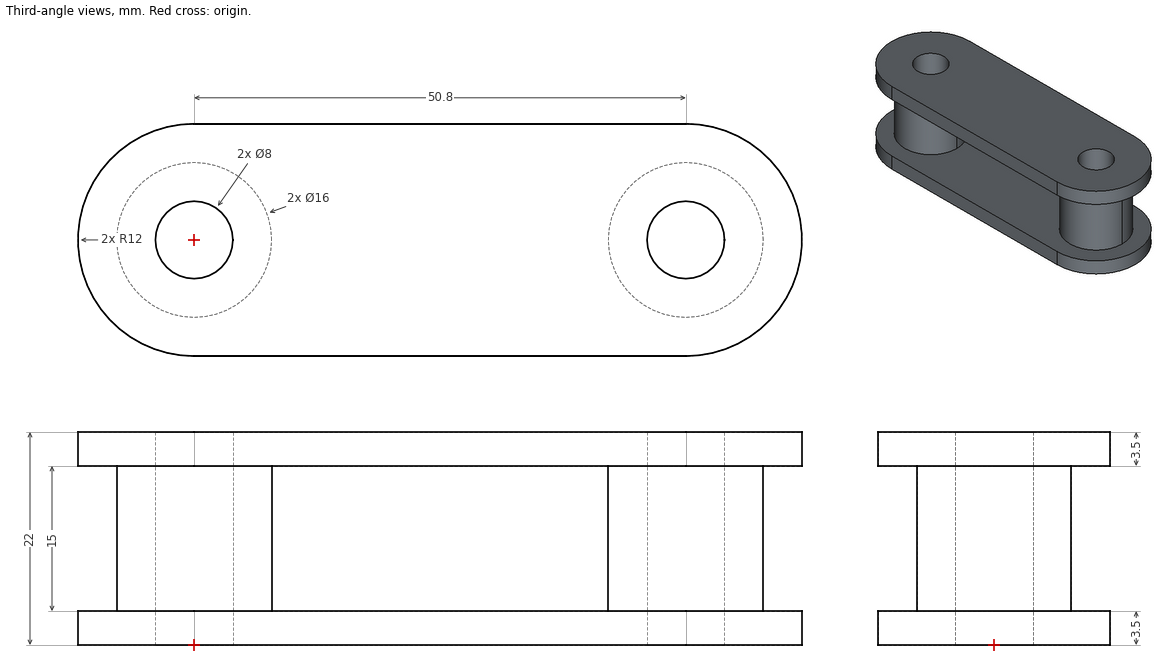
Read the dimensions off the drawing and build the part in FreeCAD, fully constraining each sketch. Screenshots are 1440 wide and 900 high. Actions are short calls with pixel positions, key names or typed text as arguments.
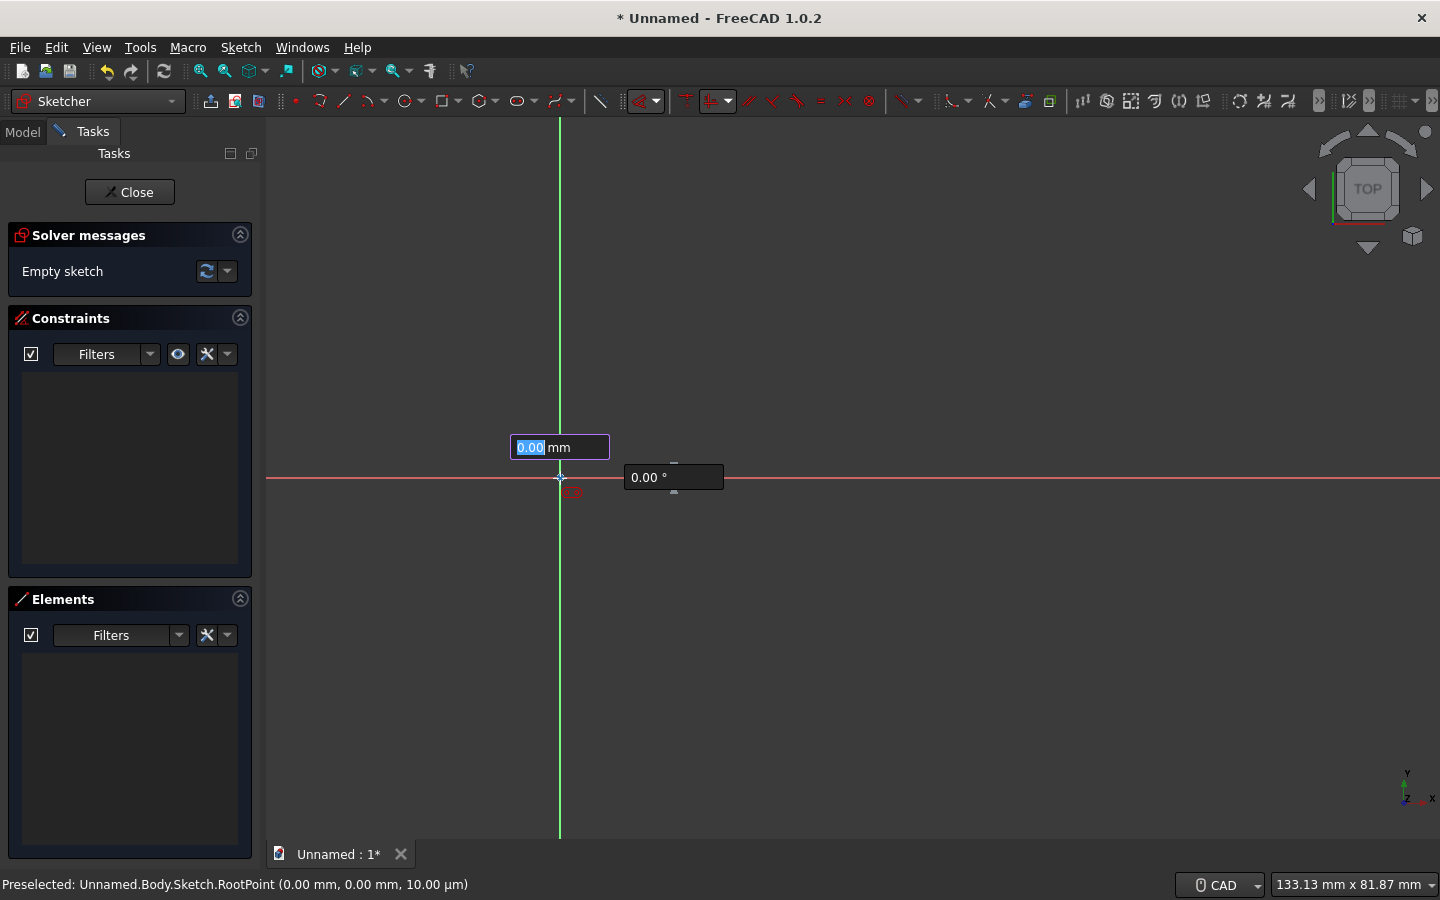
click(1008, 469)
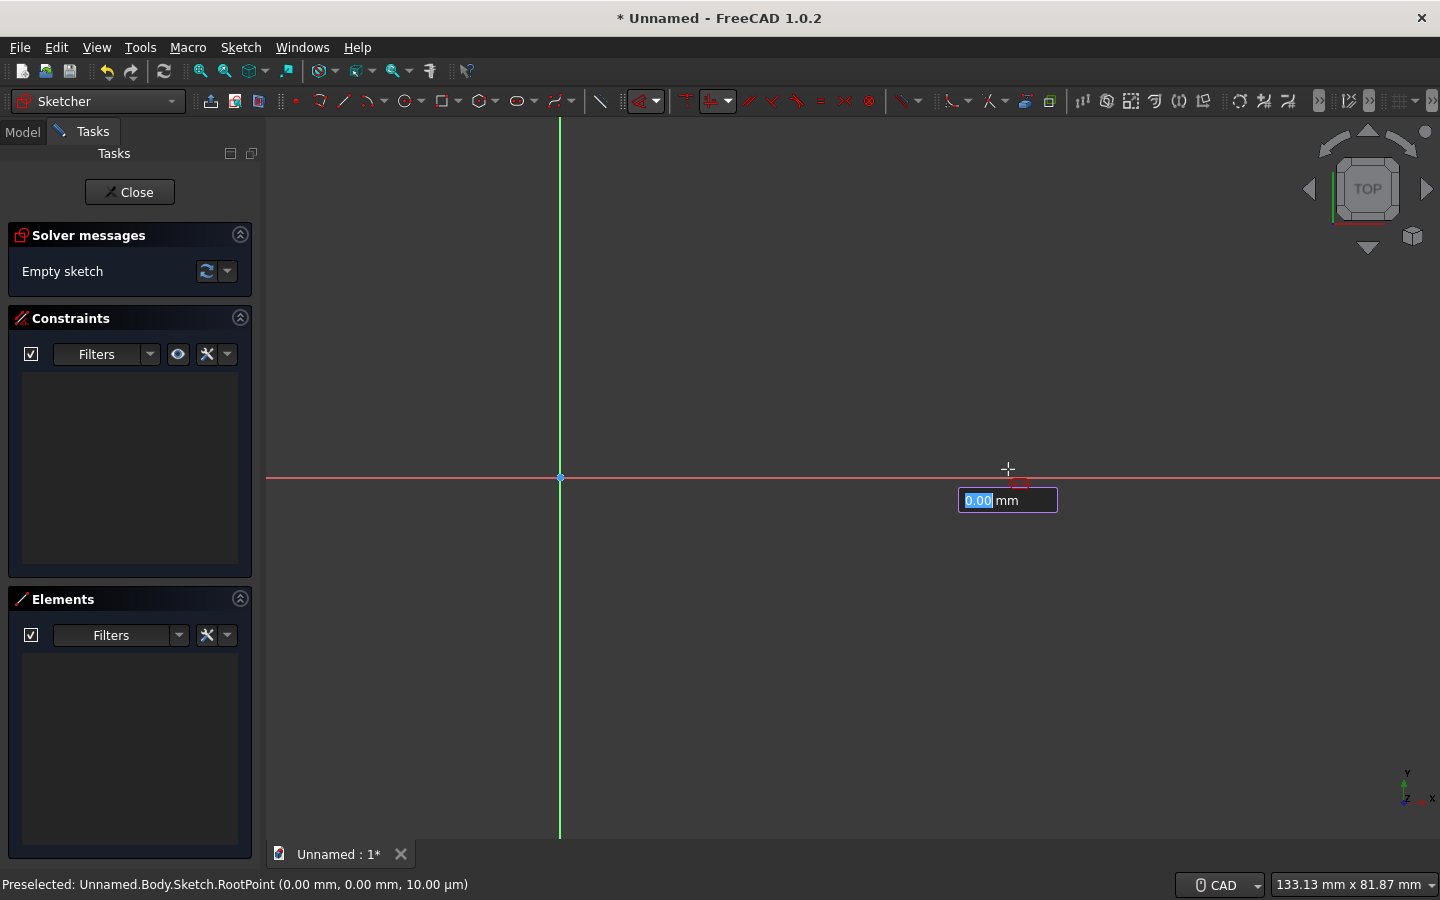
click(784, 372)
key(Escape)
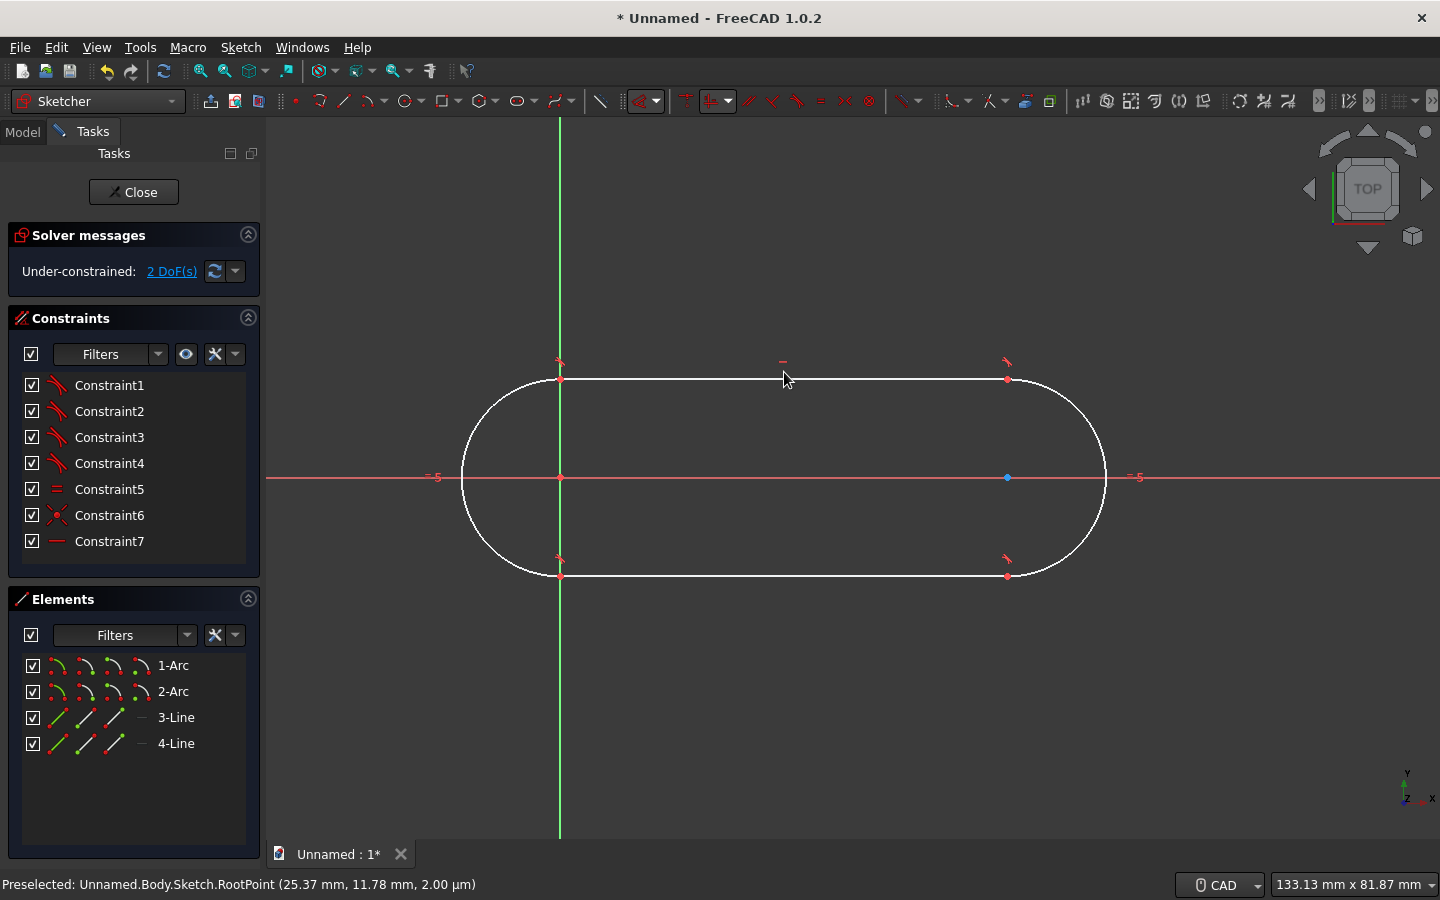
click(481, 420)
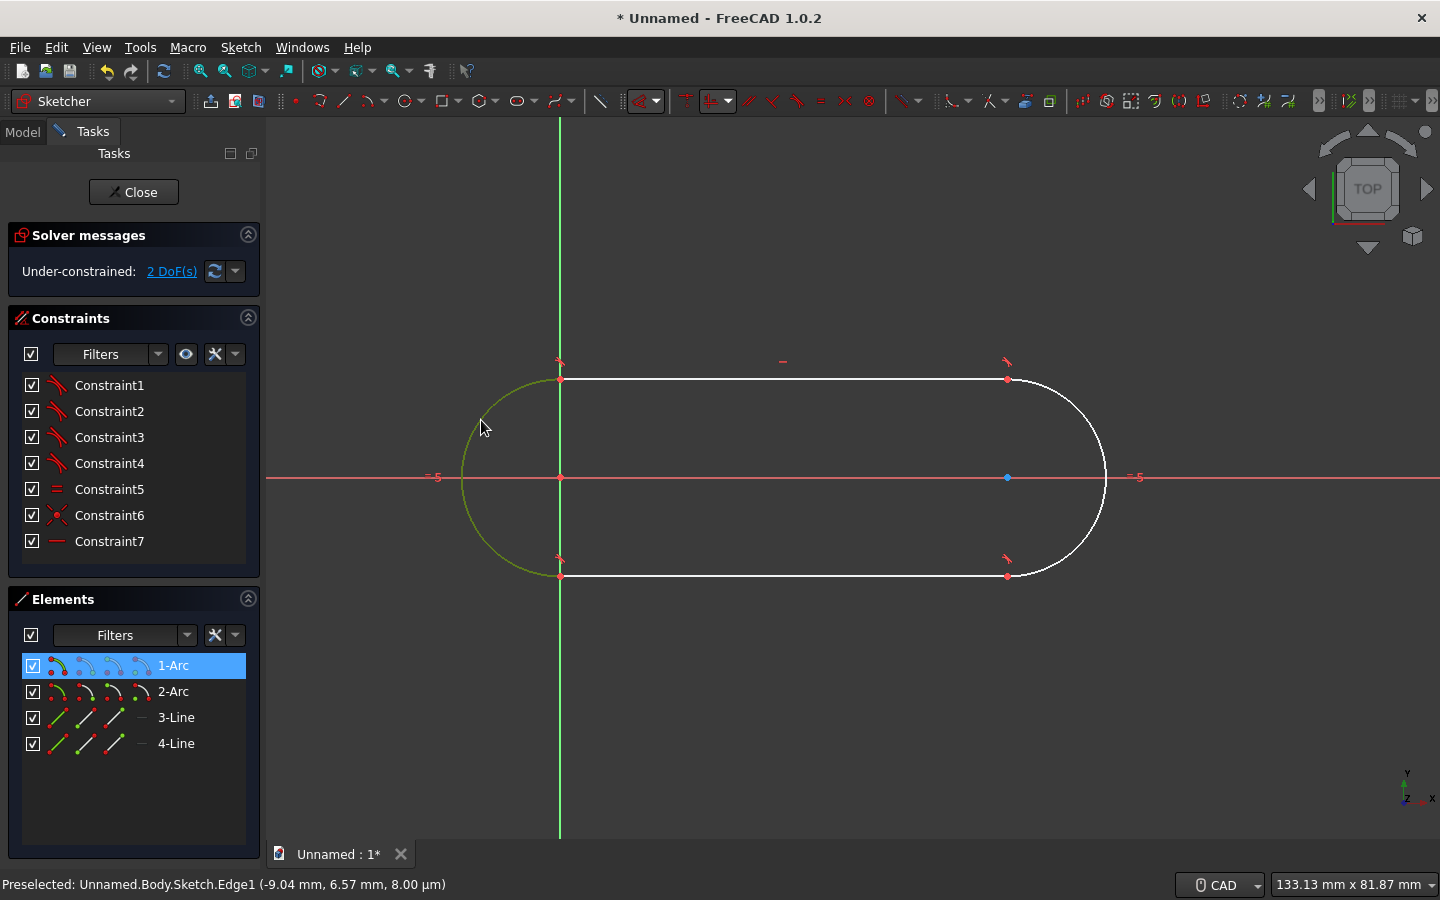
key(k)
key(r)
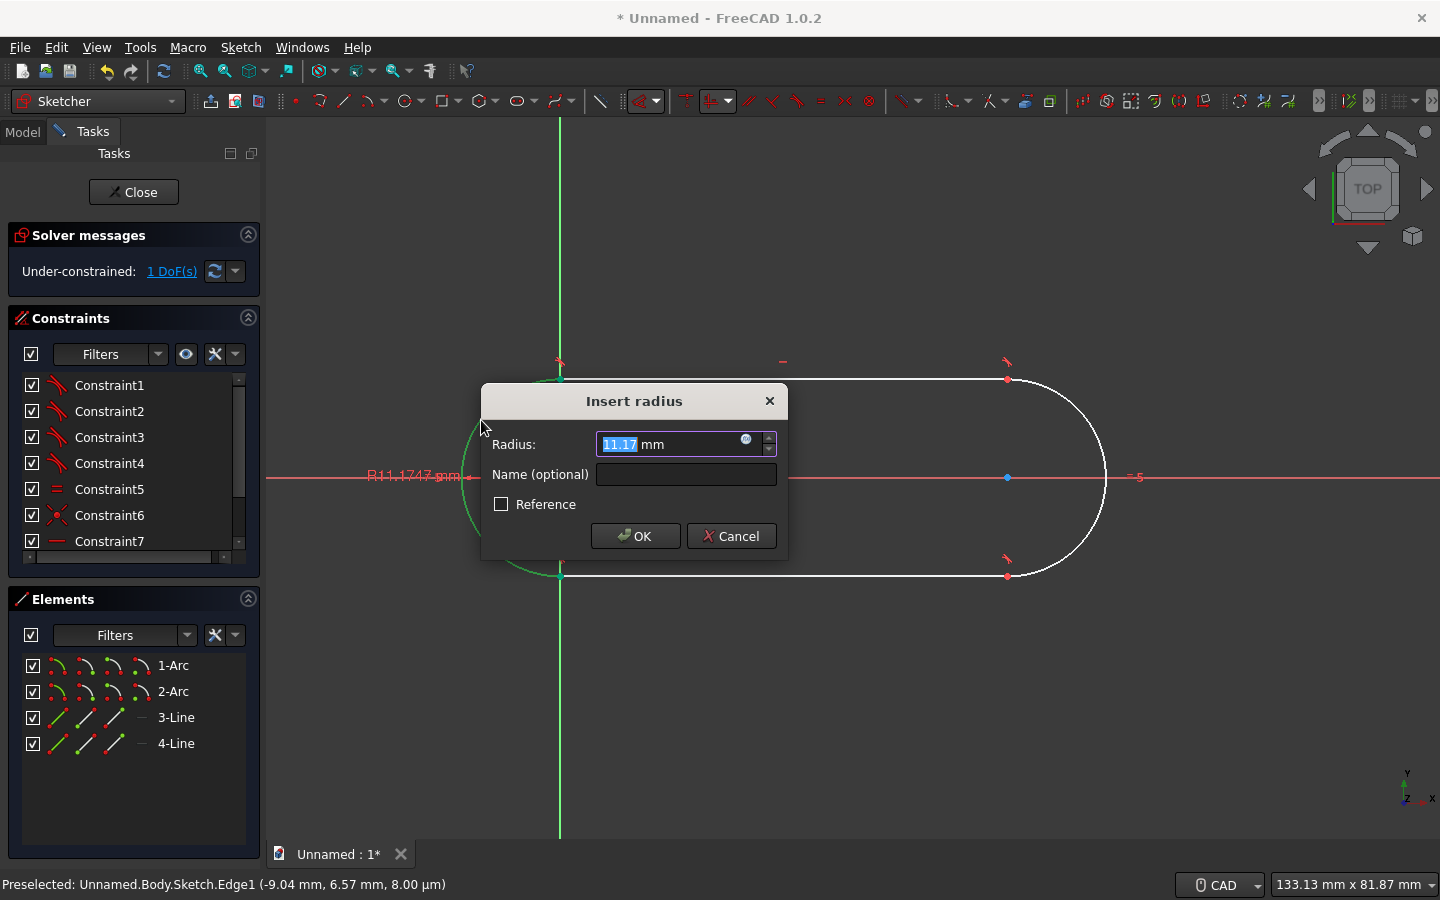
text(12)
key(Return)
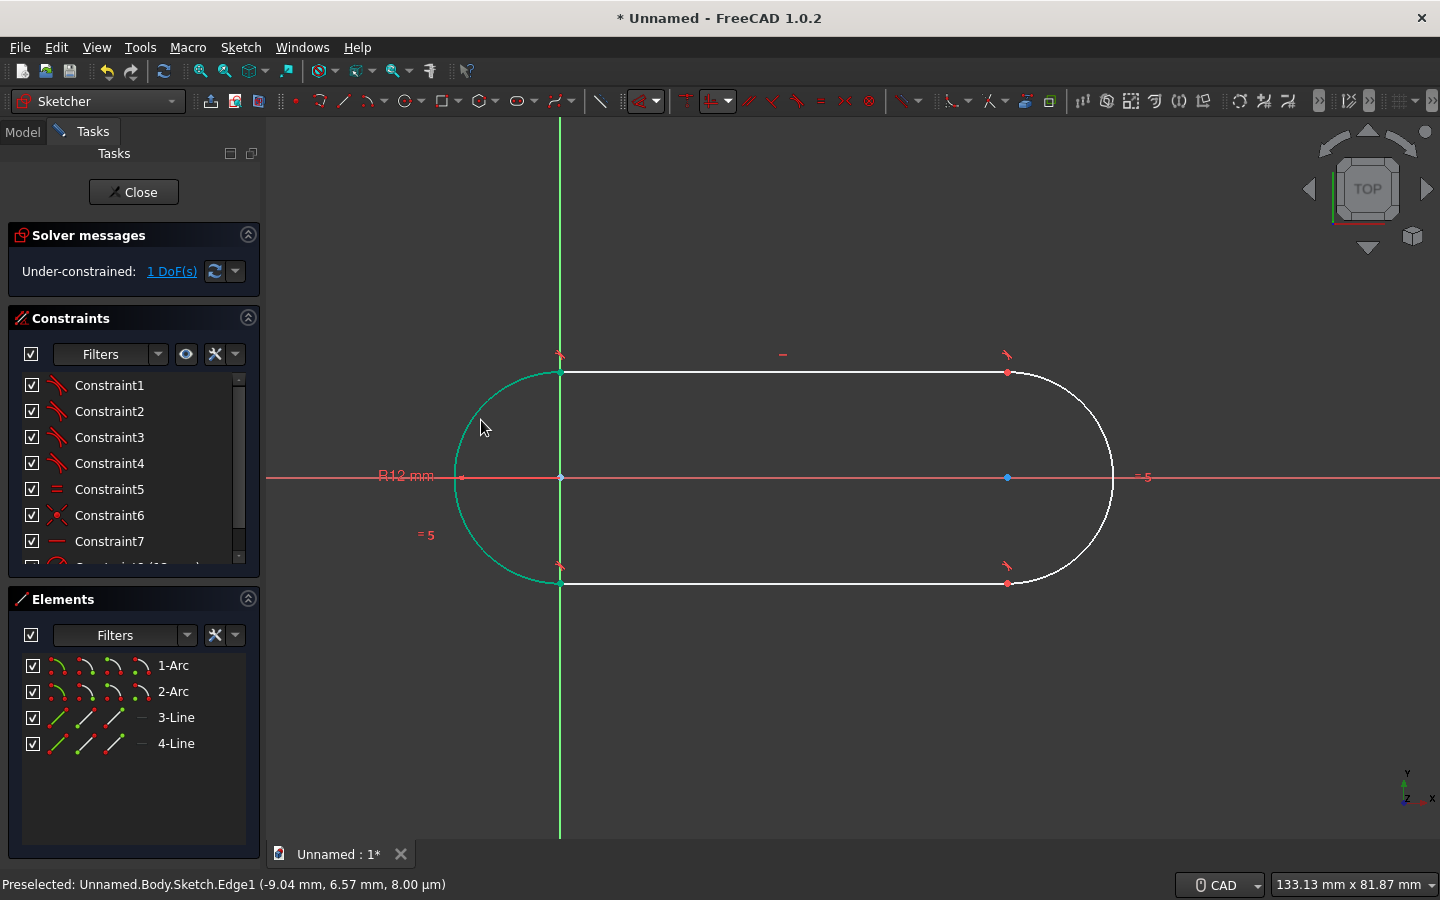
click(694, 372)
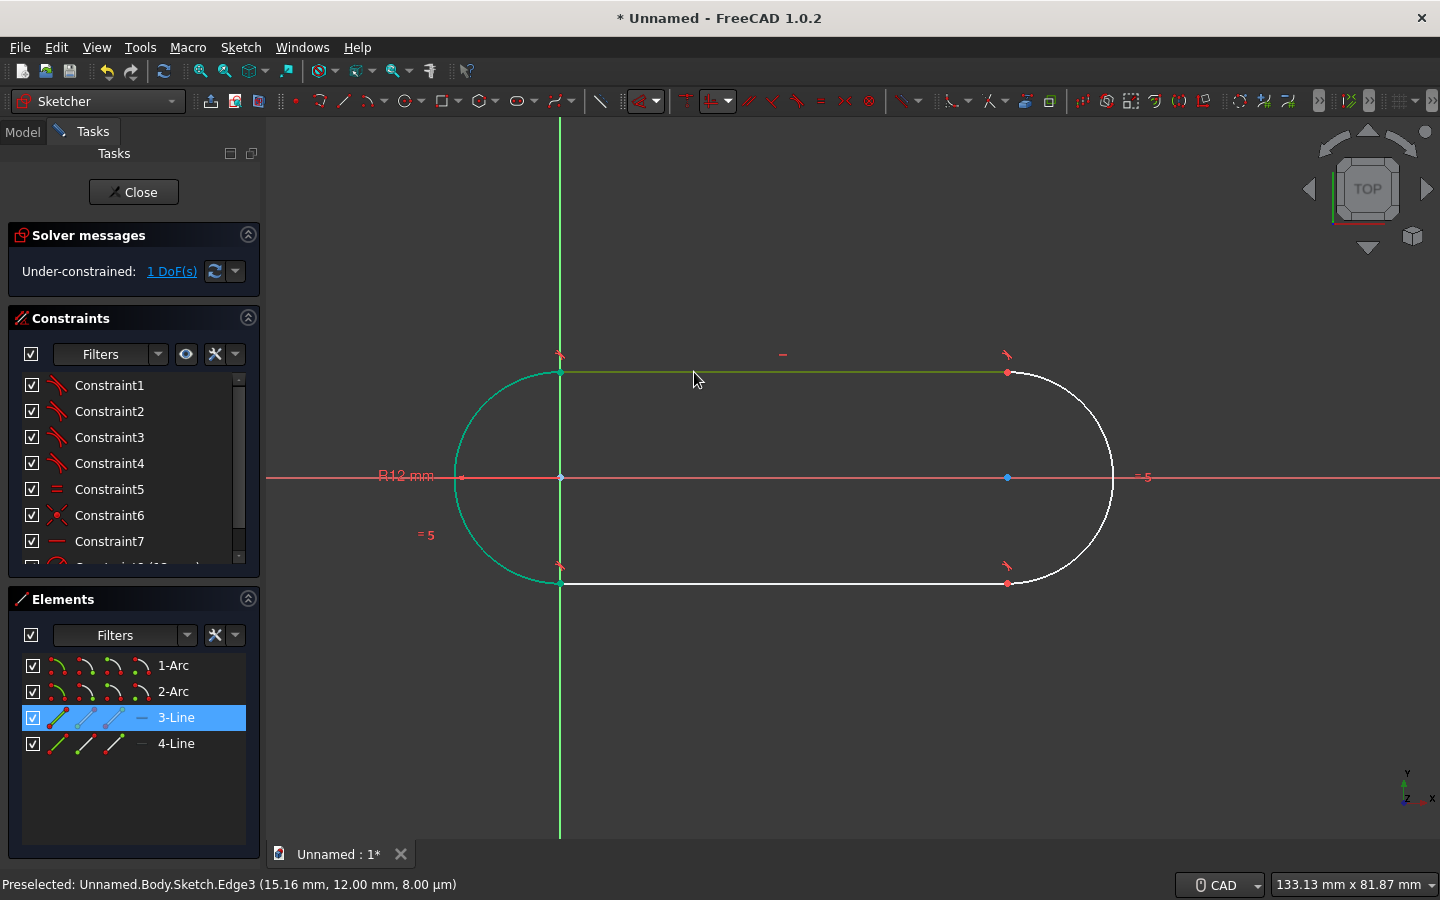
click(658, 102)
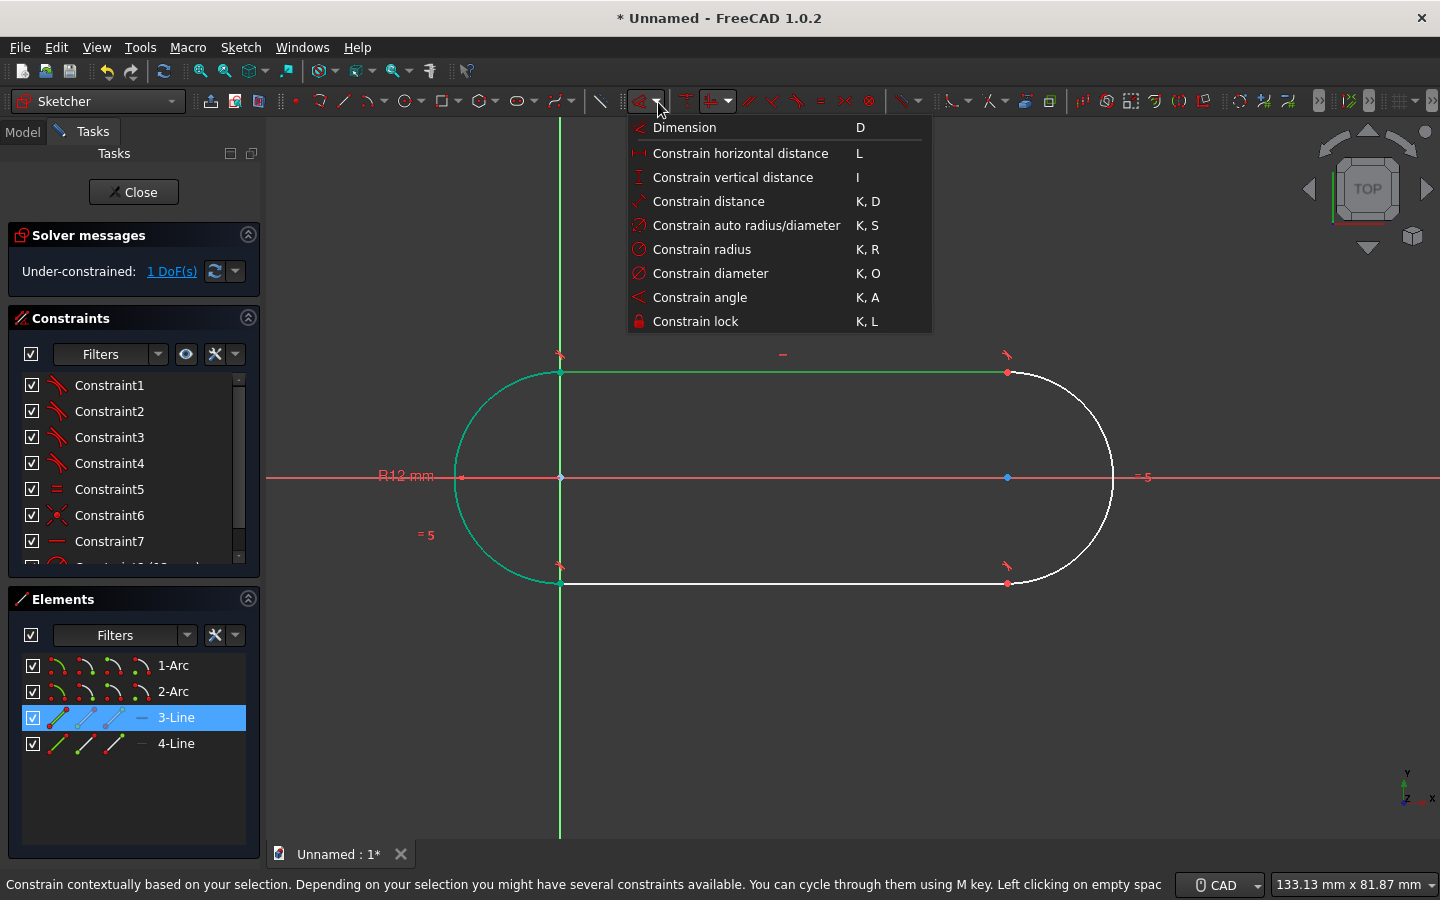
click(780, 153)